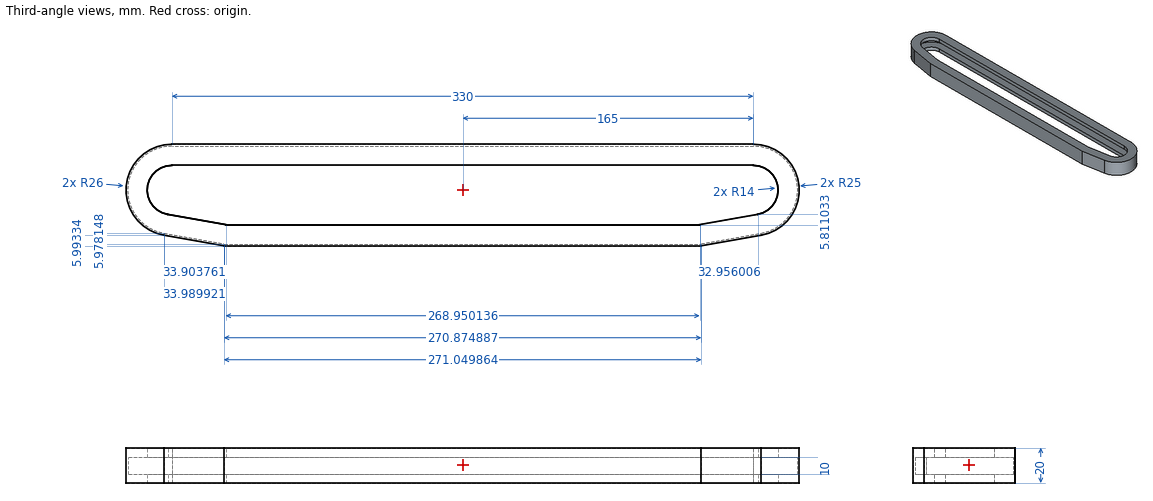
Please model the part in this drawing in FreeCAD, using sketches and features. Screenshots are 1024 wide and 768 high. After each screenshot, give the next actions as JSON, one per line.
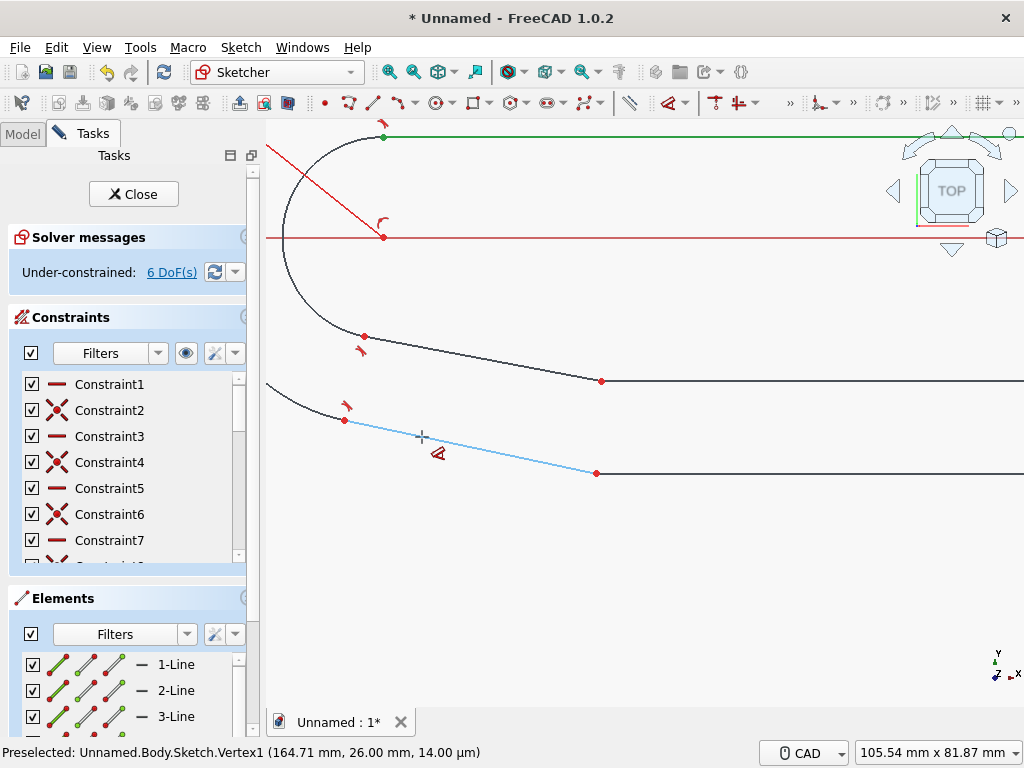
{"action": "left_click", "coordinate": [420, 436]}
{"action": "left_click", "coordinate": [310, 447]}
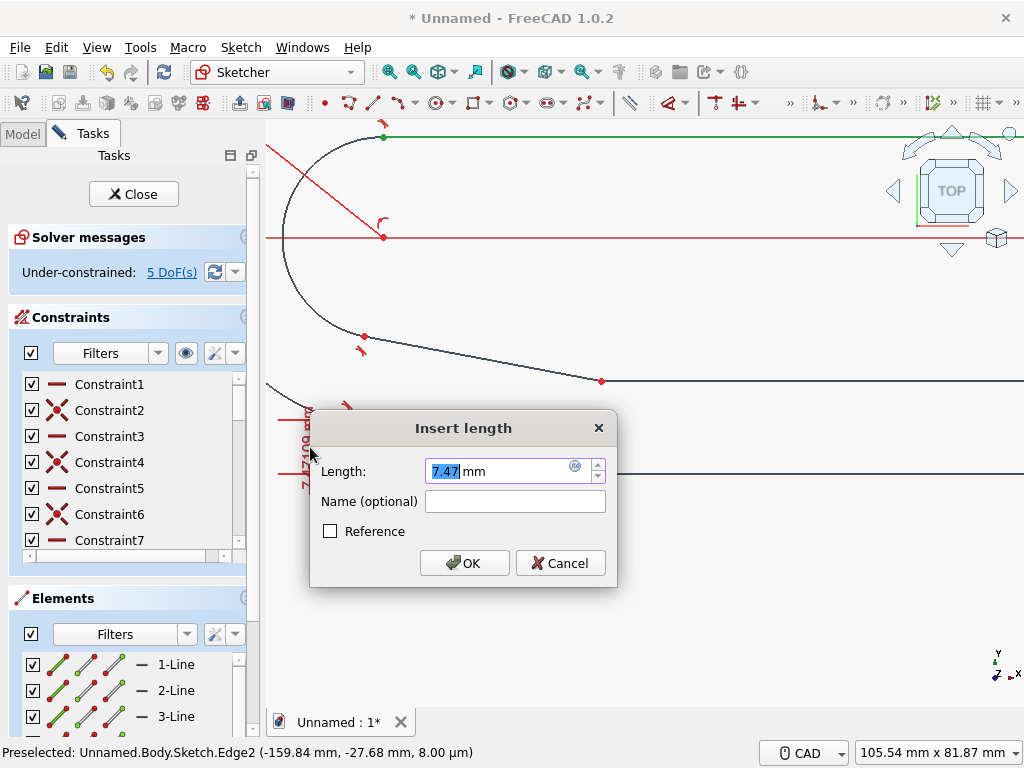
{"action": "type", "text": "5.99334"}
{"action": "key", "text": "Return"}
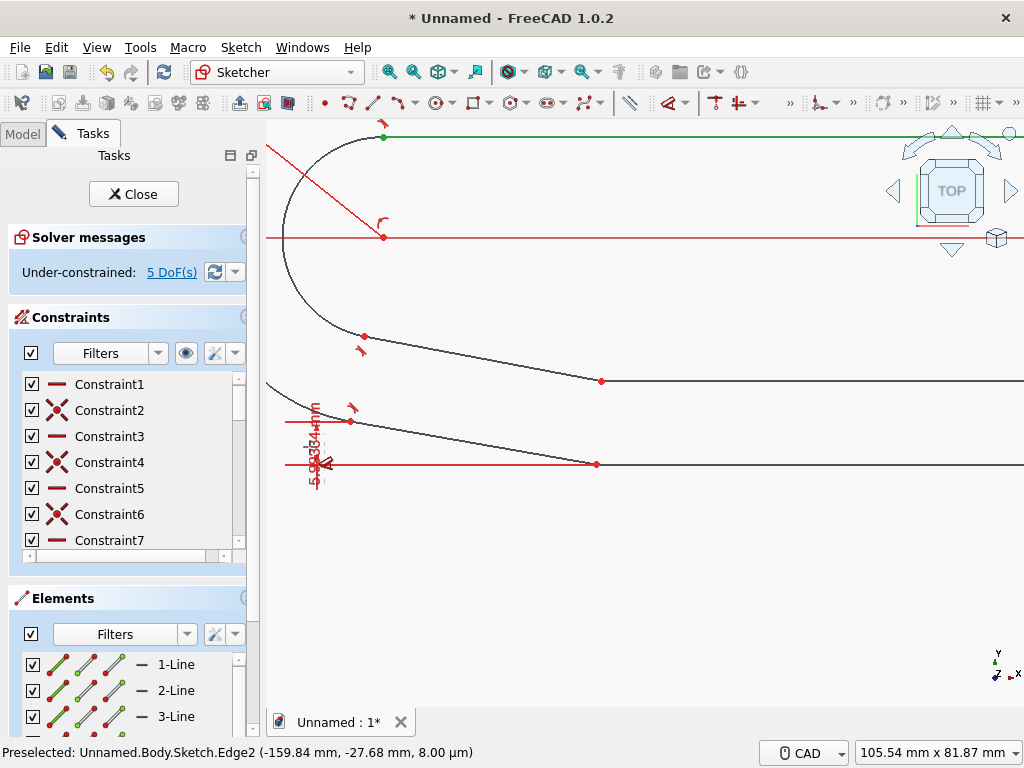
{"action": "scroll", "coordinate": [421, 437], "scroll_direction": "down", "scroll_amount": 10}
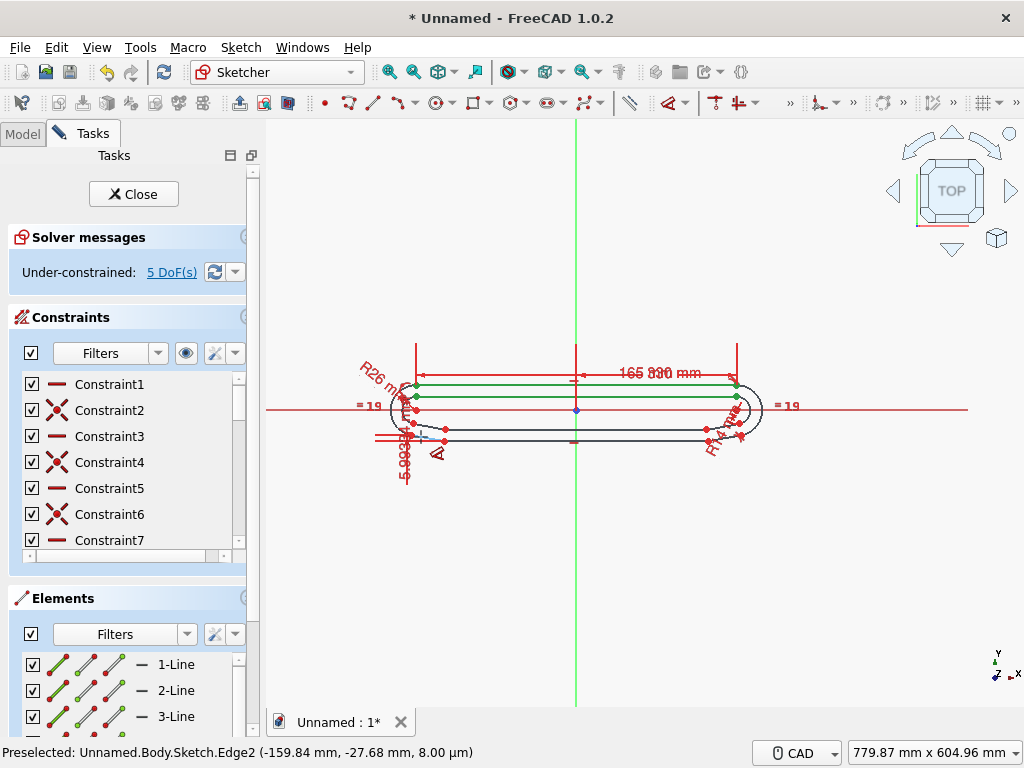
{"action": "scroll", "coordinate": [730, 426], "scroll_direction": "up", "scroll_amount": 10}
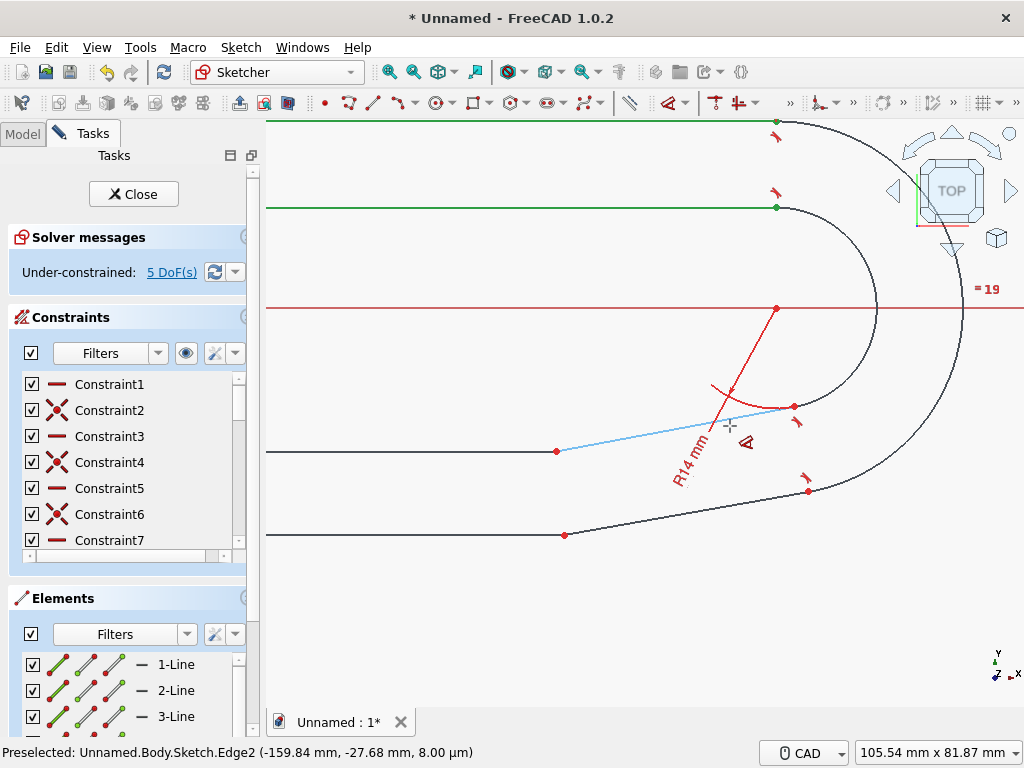
{"action": "left_click", "coordinate": [723, 420]}
{"action": "left_click", "coordinate": [829, 429]}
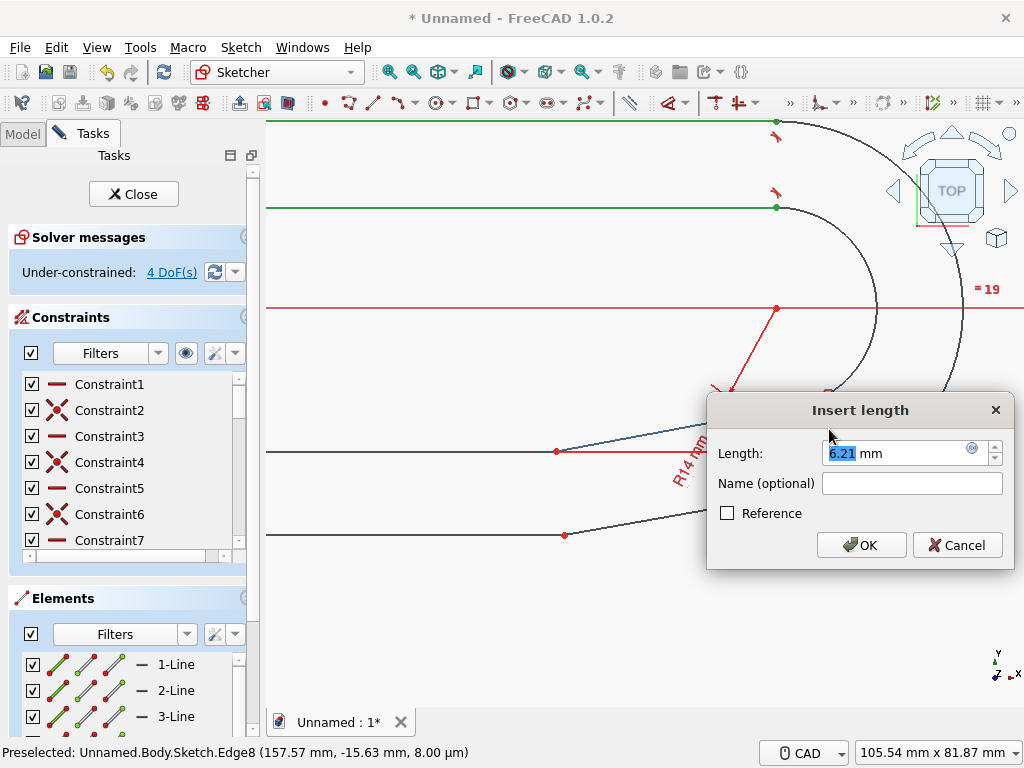
{"action": "type", "text": "5.811033"}
{"action": "key", "text": "Return"}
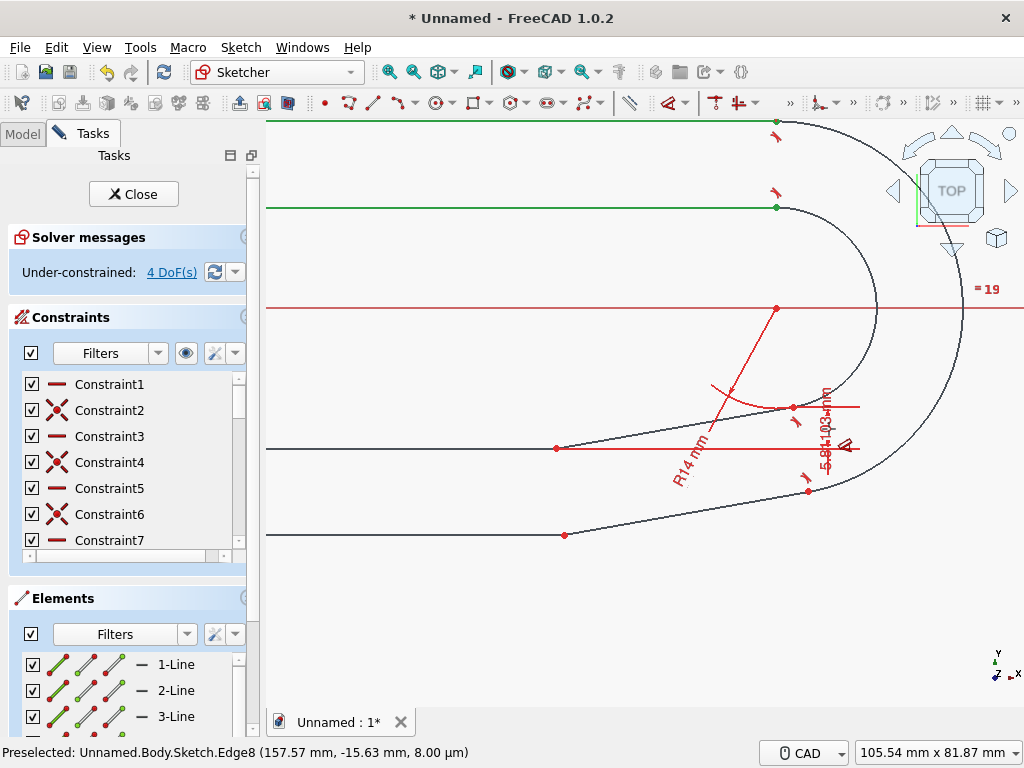
{"action": "scroll", "coordinate": [731, 426], "scroll_direction": "down", "scroll_amount": 10}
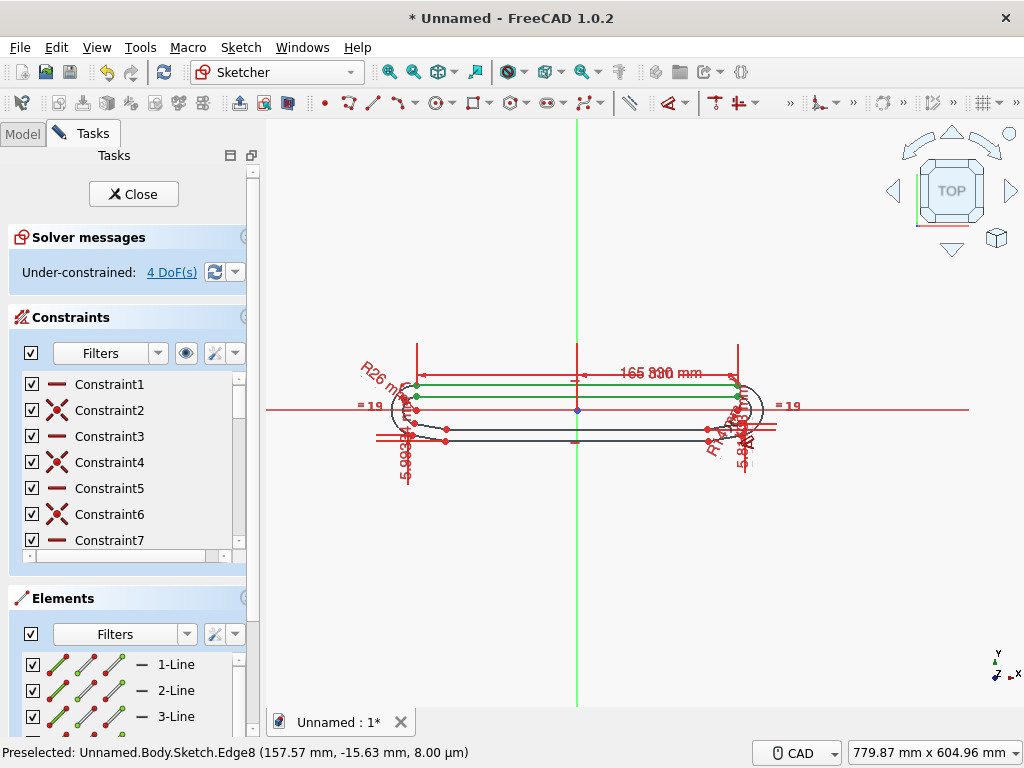
{"action": "left_click", "coordinate": [525, 441]}
{"action": "left_click", "coordinate": [517, 475]}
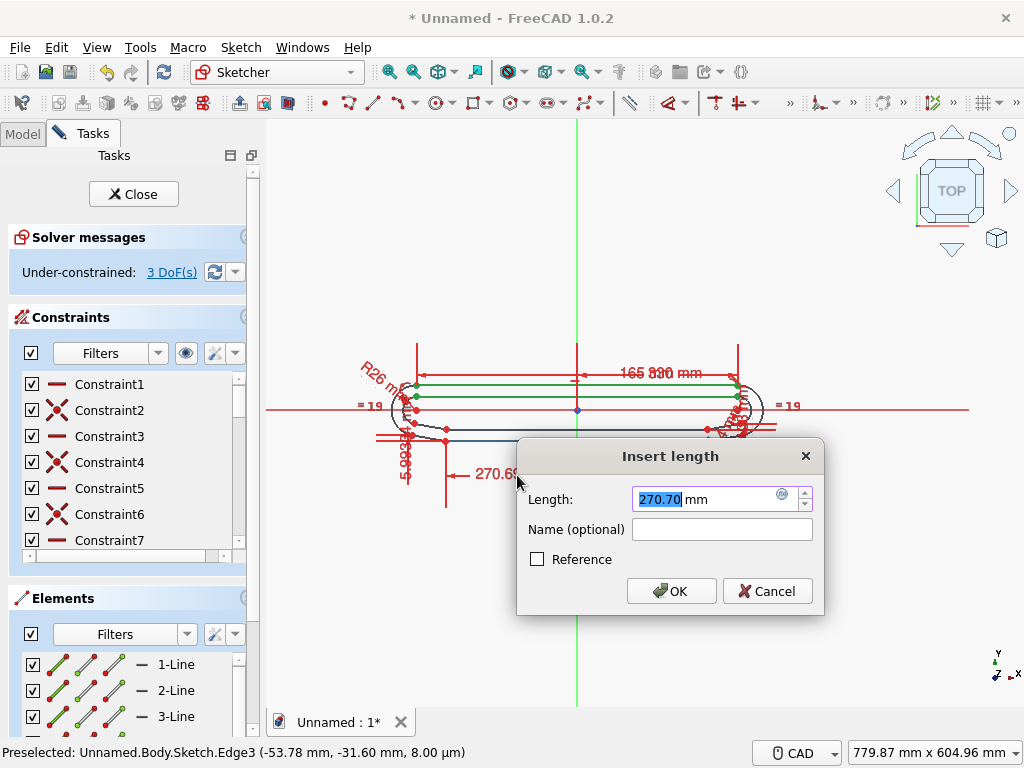
{"action": "type", "text": "271.049864"}
{"action": "key", "text": "Return"}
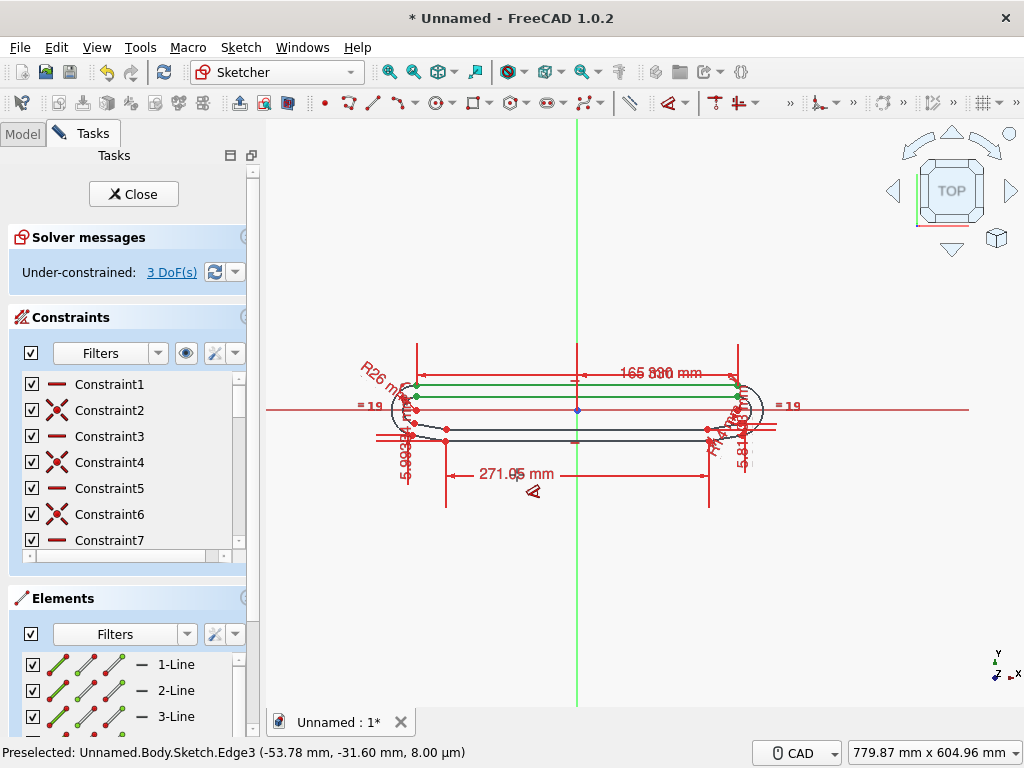
{"action": "left_click", "coordinate": [629, 430]}
{"action": "left_click", "coordinate": [637, 464]}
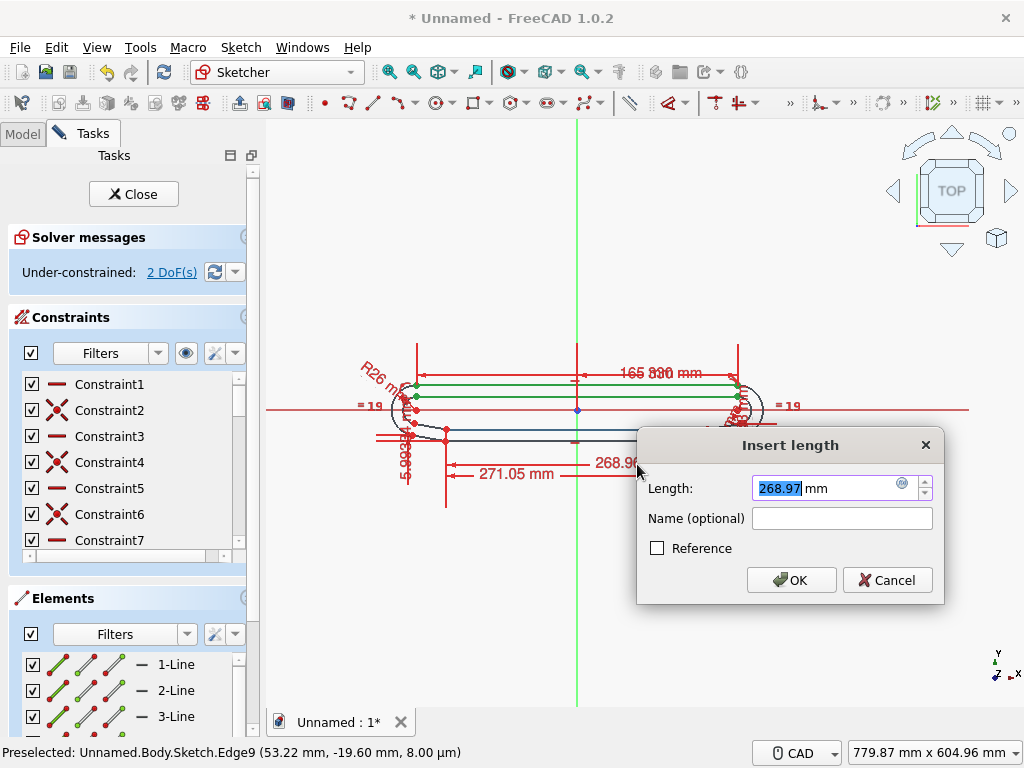
{"action": "type", "text": "268.950136"}
{"action": "key", "text": "Return"}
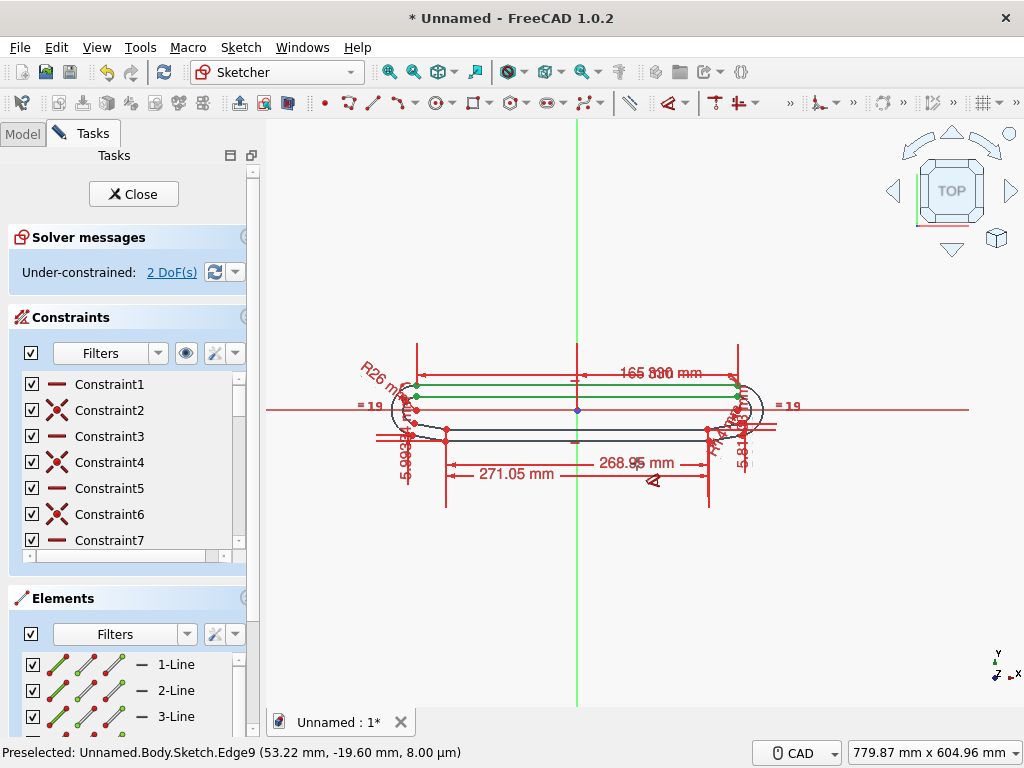
{"action": "scroll", "coordinate": [422, 437], "scroll_direction": "up", "scroll_amount": 2}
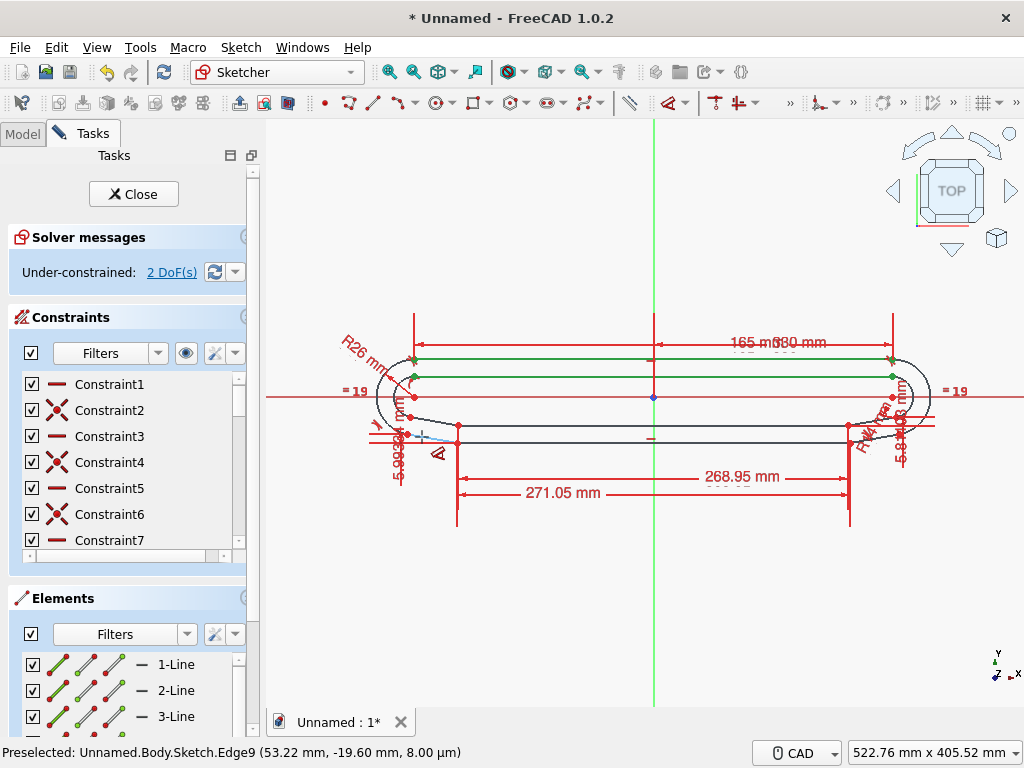
{"action": "left_click", "coordinate": [423, 437]}
{"action": "left_click", "coordinate": [432, 477]}